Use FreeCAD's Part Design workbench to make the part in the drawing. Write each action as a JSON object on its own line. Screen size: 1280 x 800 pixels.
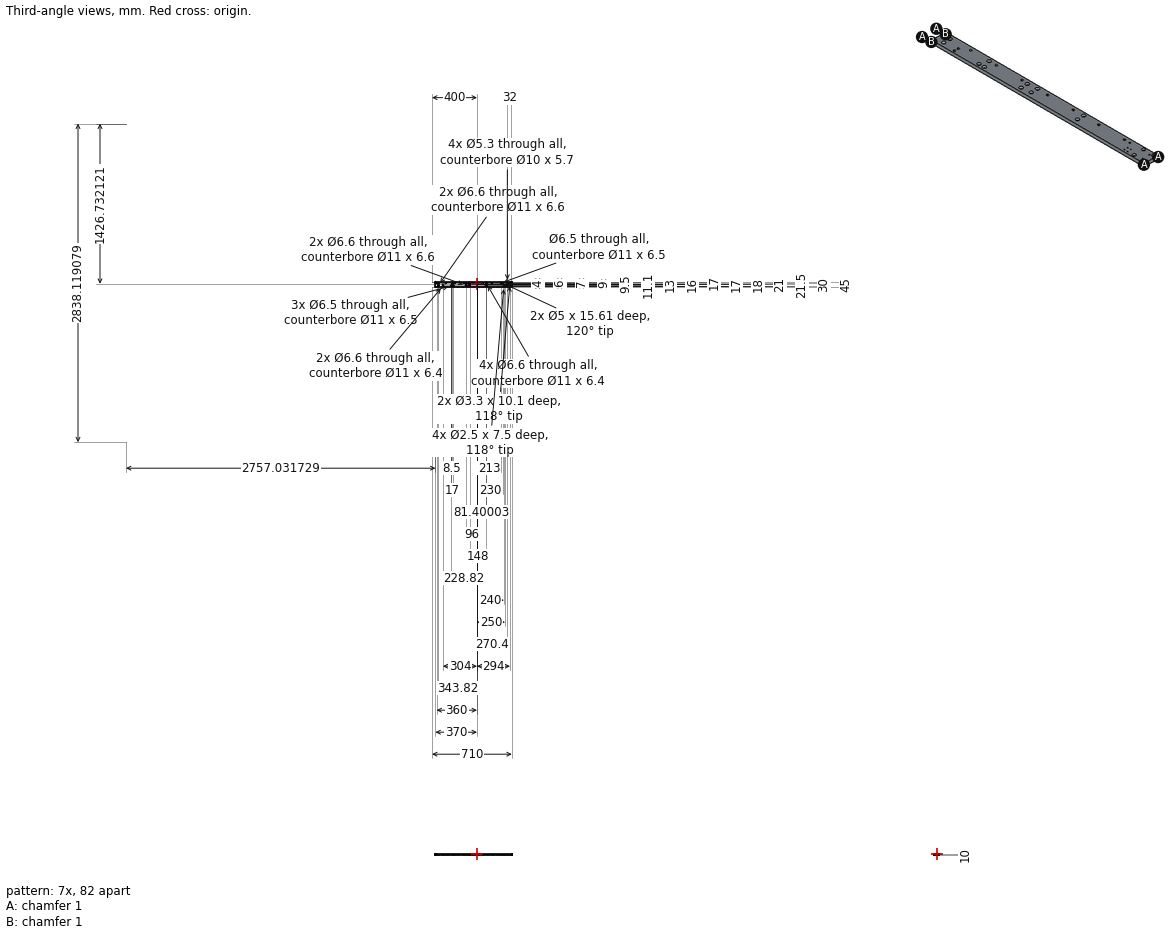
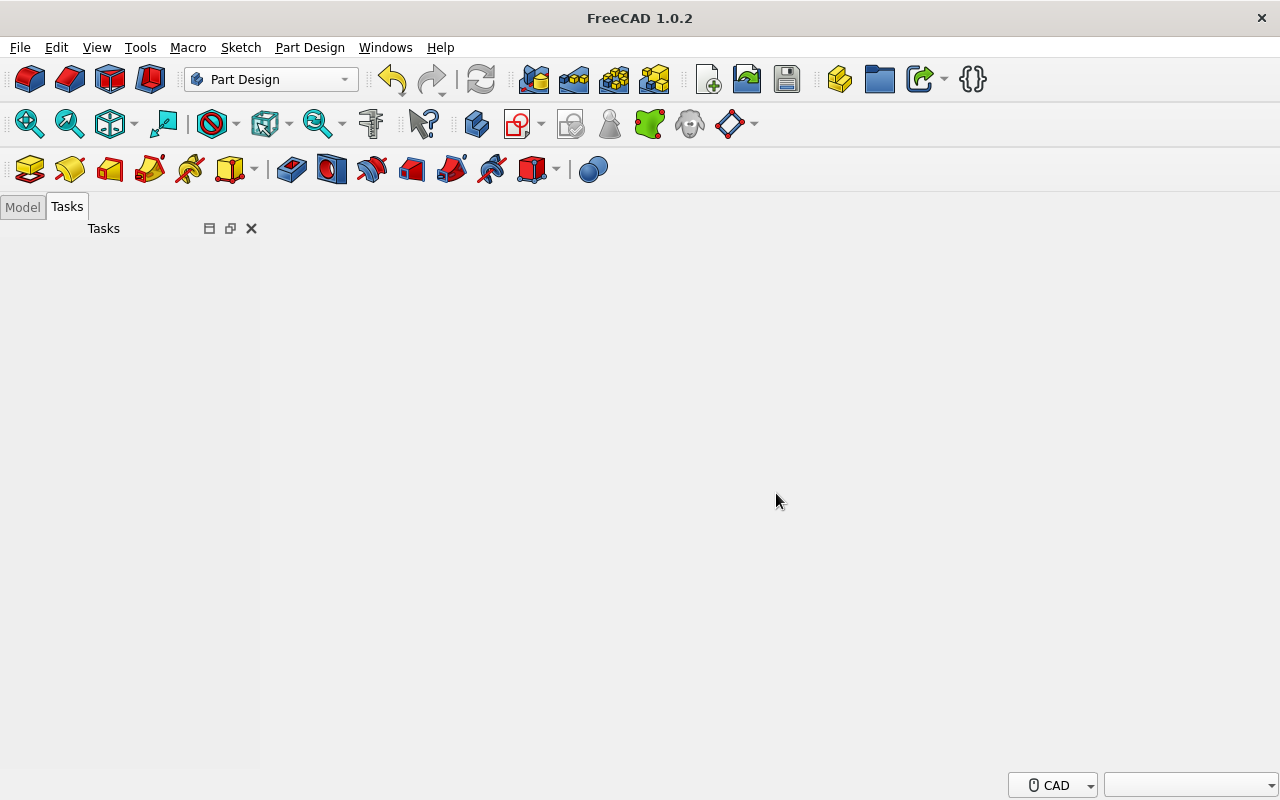
{"action": "left_click", "coordinate": [708, 80]}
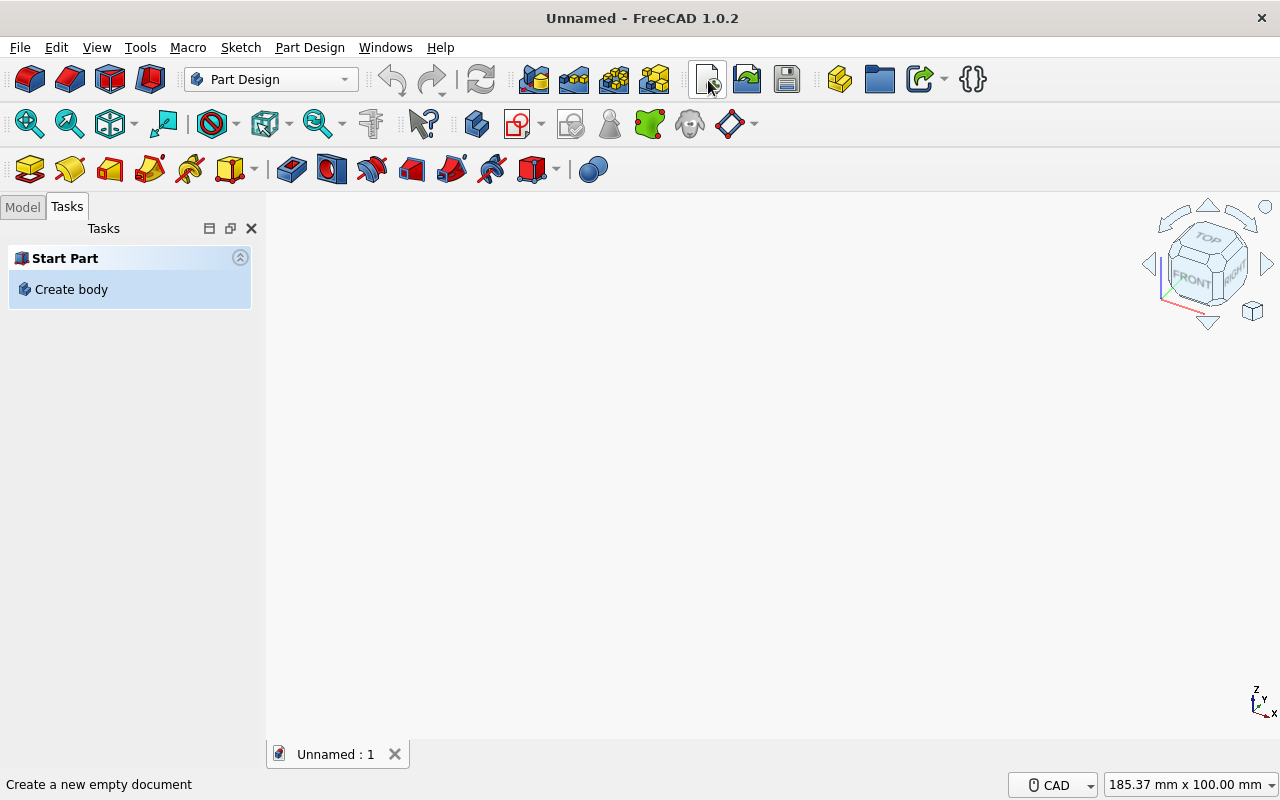
{"action": "left_click", "coordinate": [518, 124]}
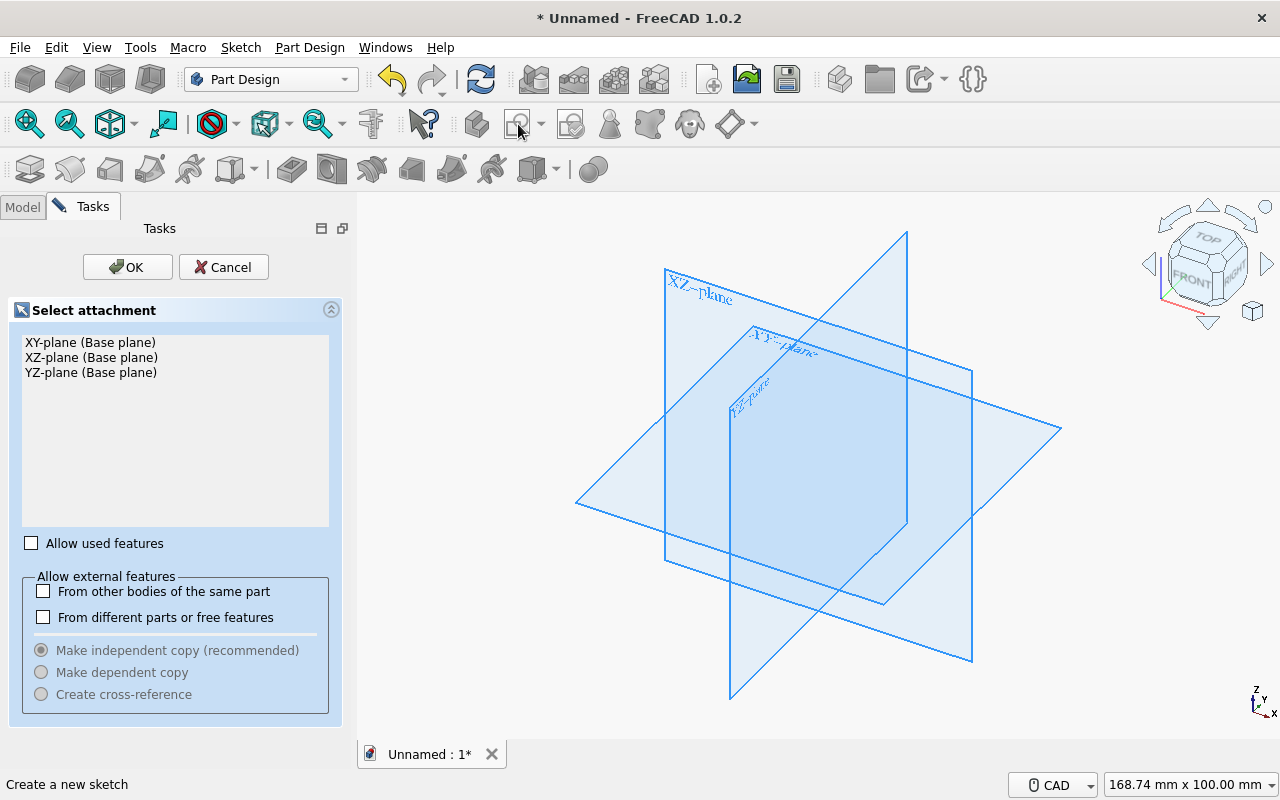
{"action": "left_click", "coordinate": [82, 342]}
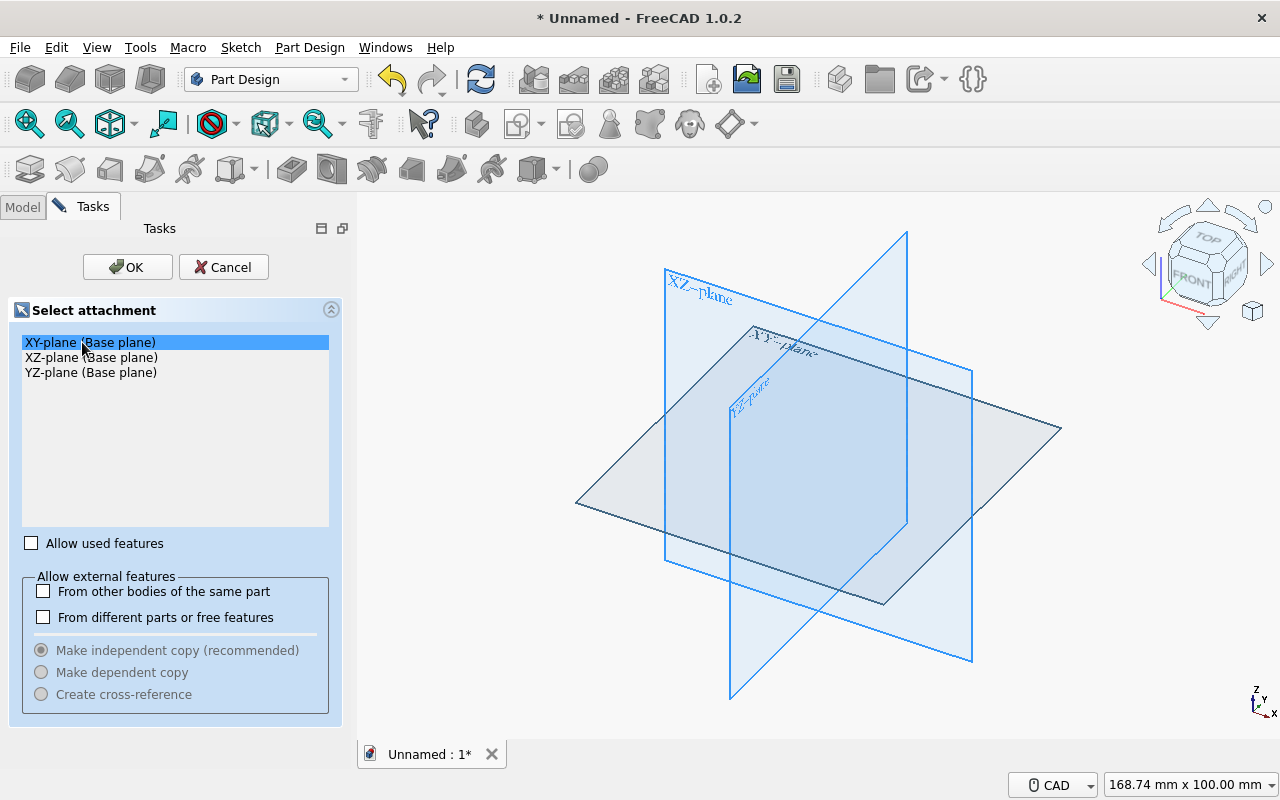
{"action": "left_click", "coordinate": [128, 267]}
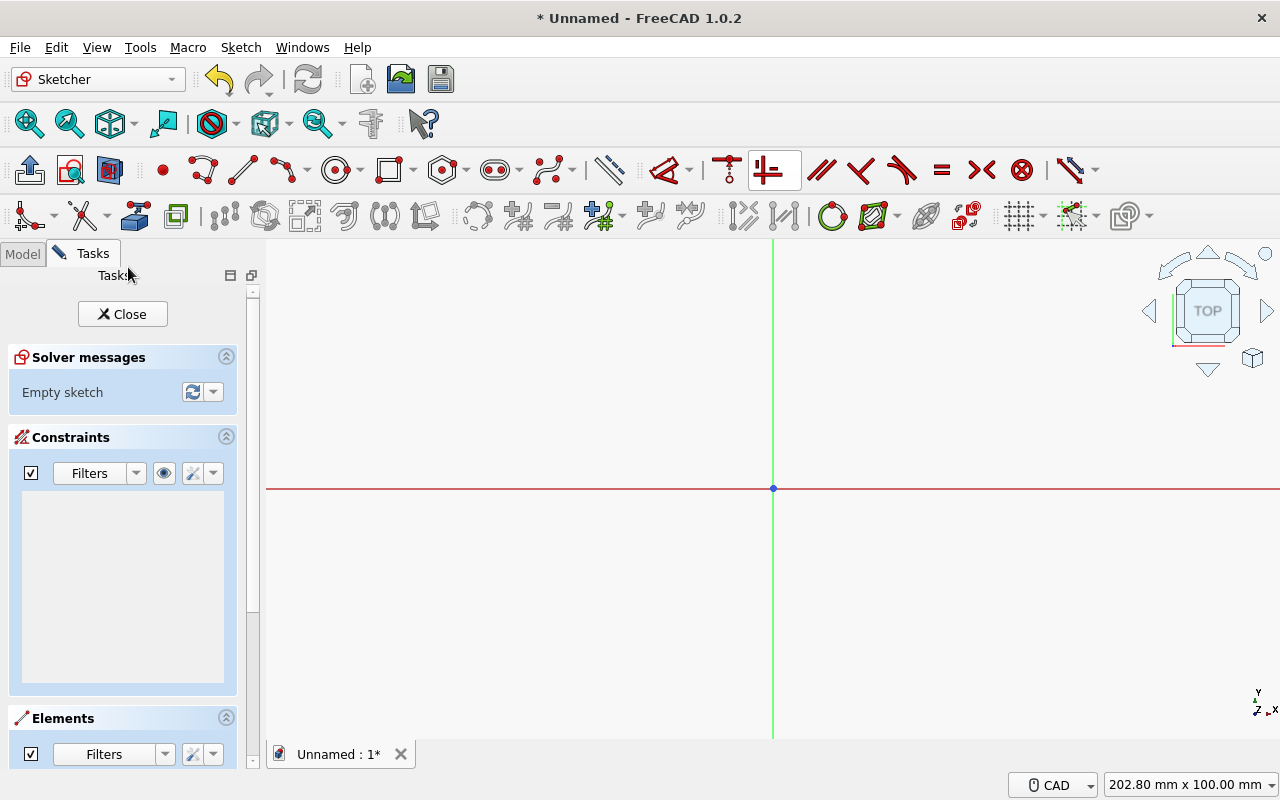
{"action": "scroll", "coordinate": [735, 484], "scroll_direction": "down", "scroll_amount": 9}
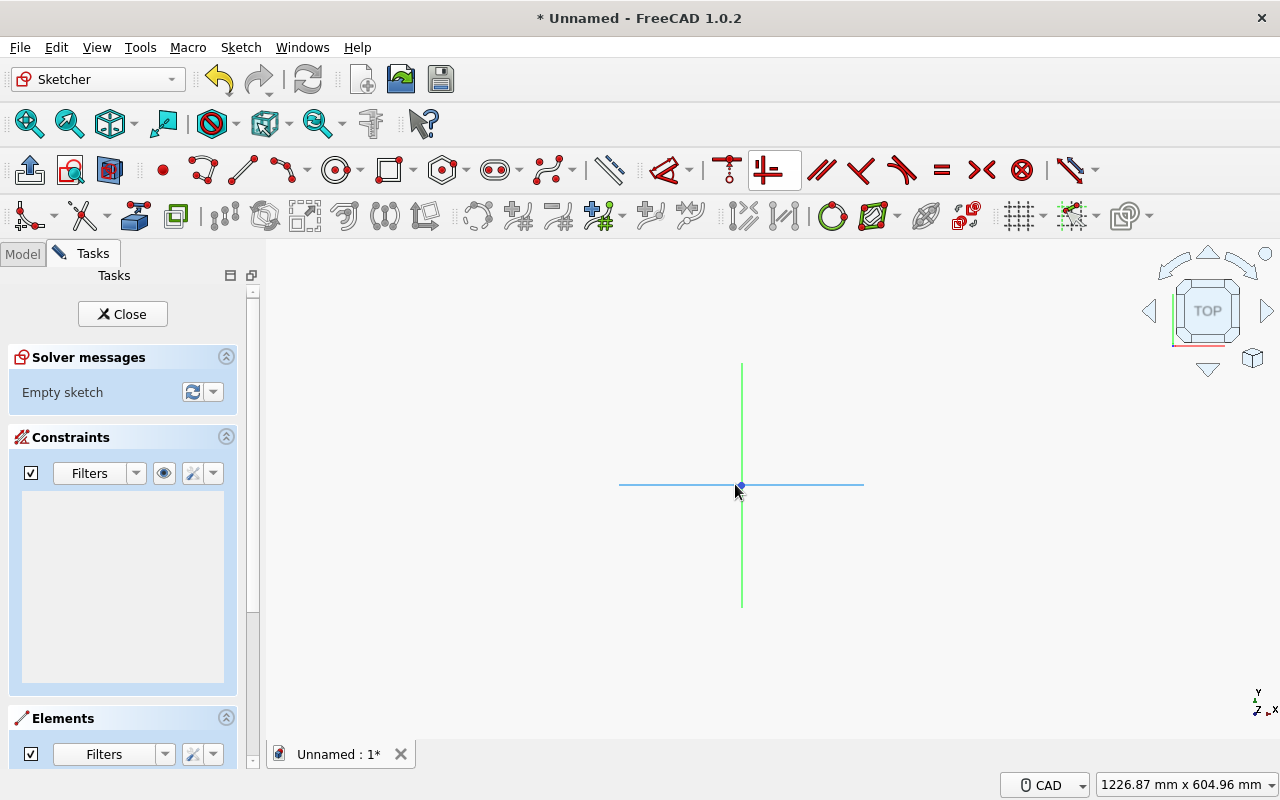
{"action": "left_click", "coordinate": [390, 170]}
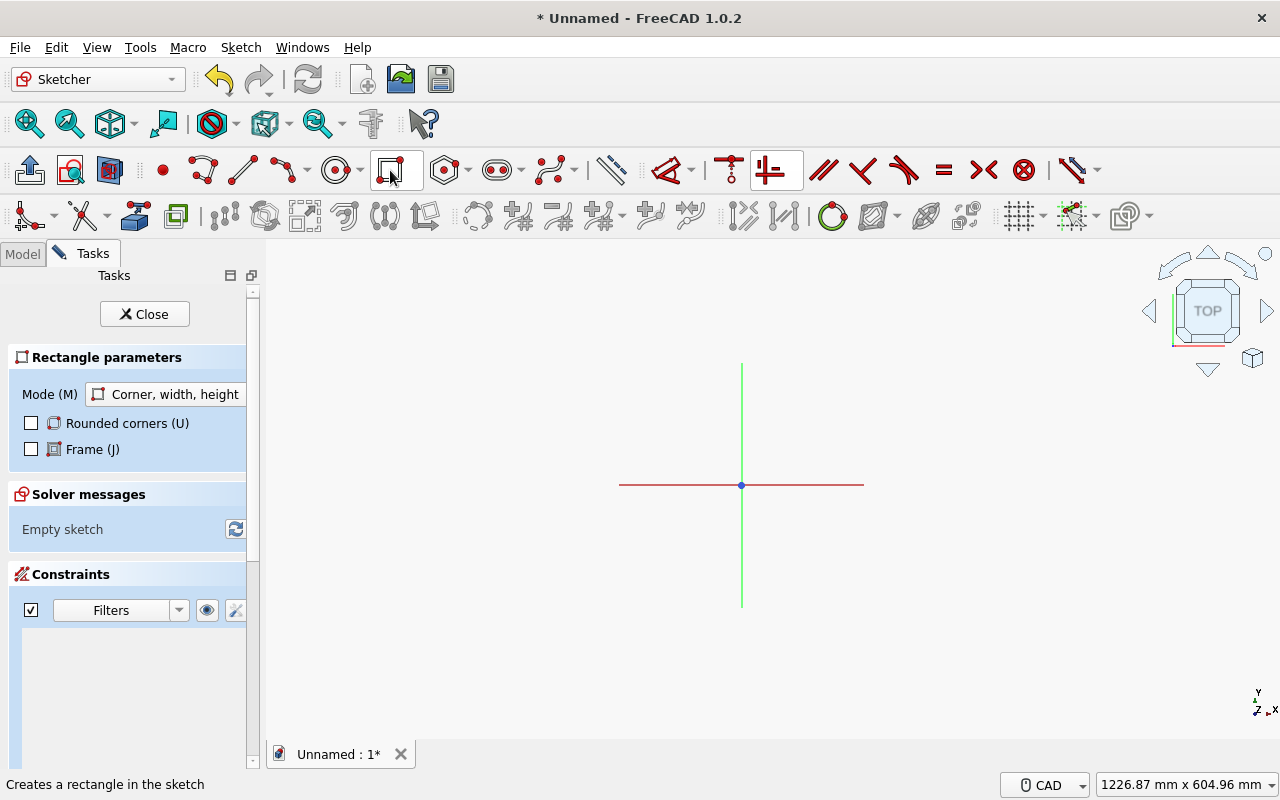
{"action": "left_click", "coordinate": [411, 471]}
{"action": "left_click", "coordinate": [998, 508]}
{"action": "key", "text": "Escape"}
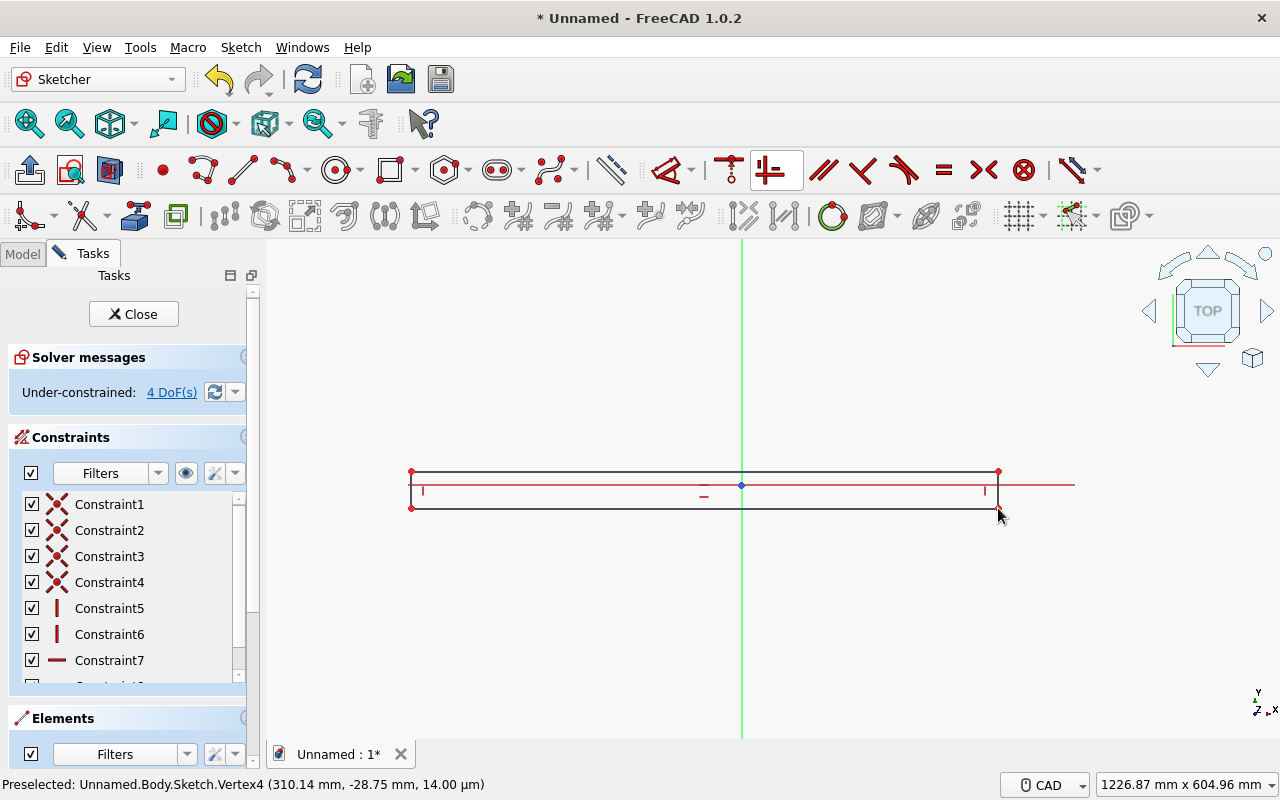
{"action": "scroll", "coordinate": [411, 483], "scroll_direction": "up", "scroll_amount": 2}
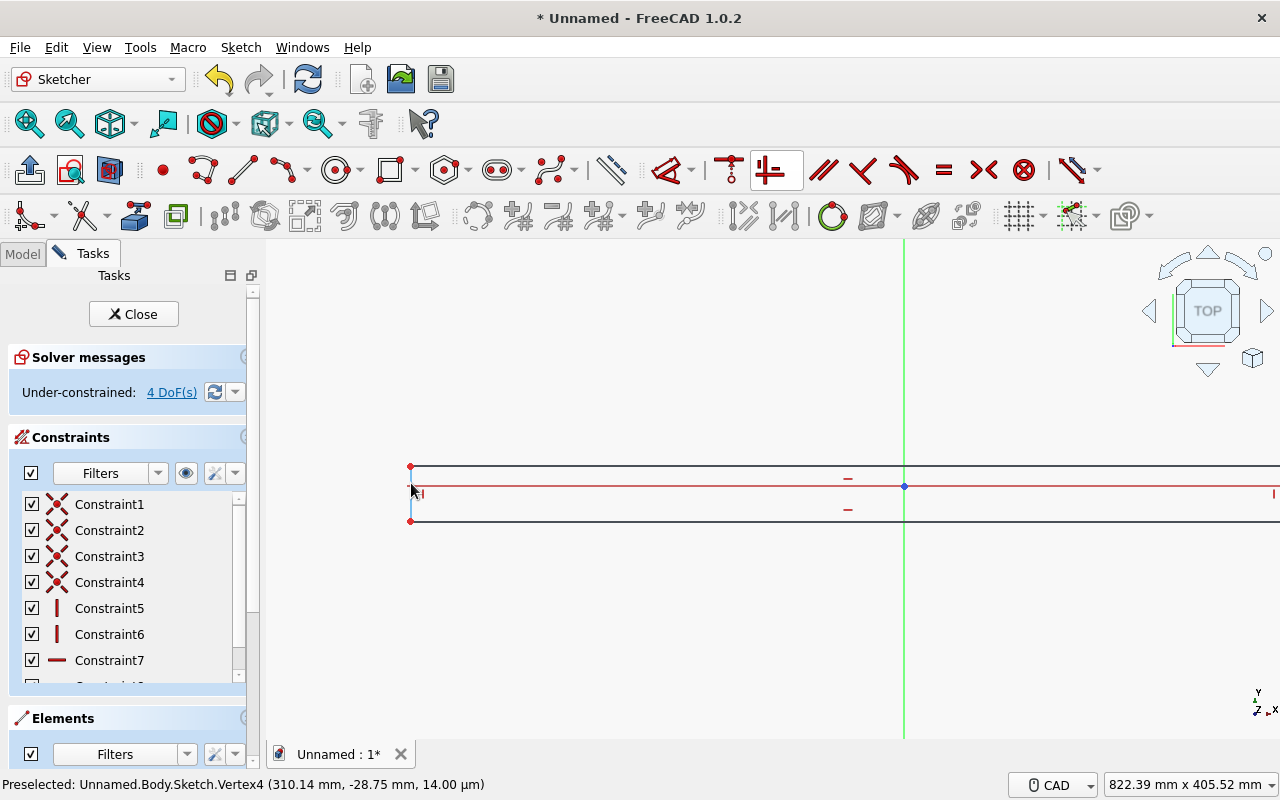
{"action": "left_click", "coordinate": [411, 483]}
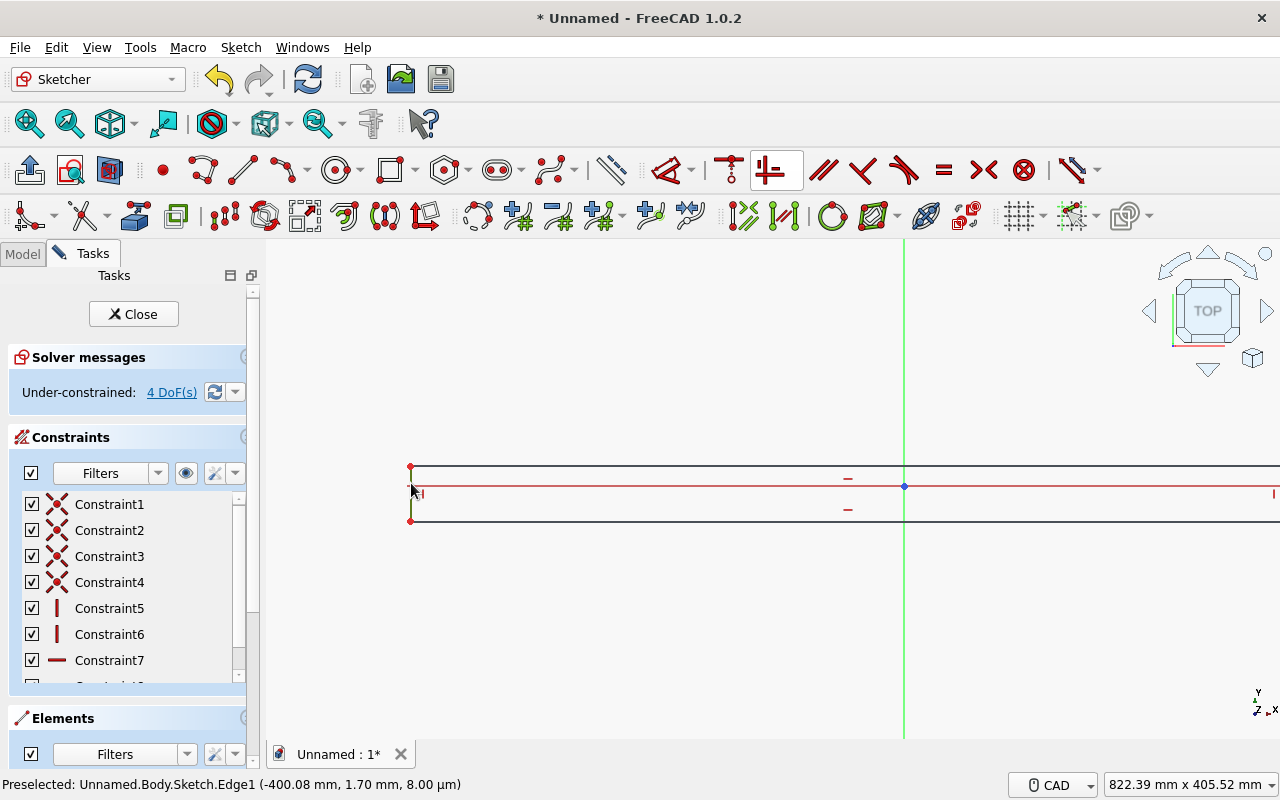
{"action": "left_click", "coordinate": [694, 170]}